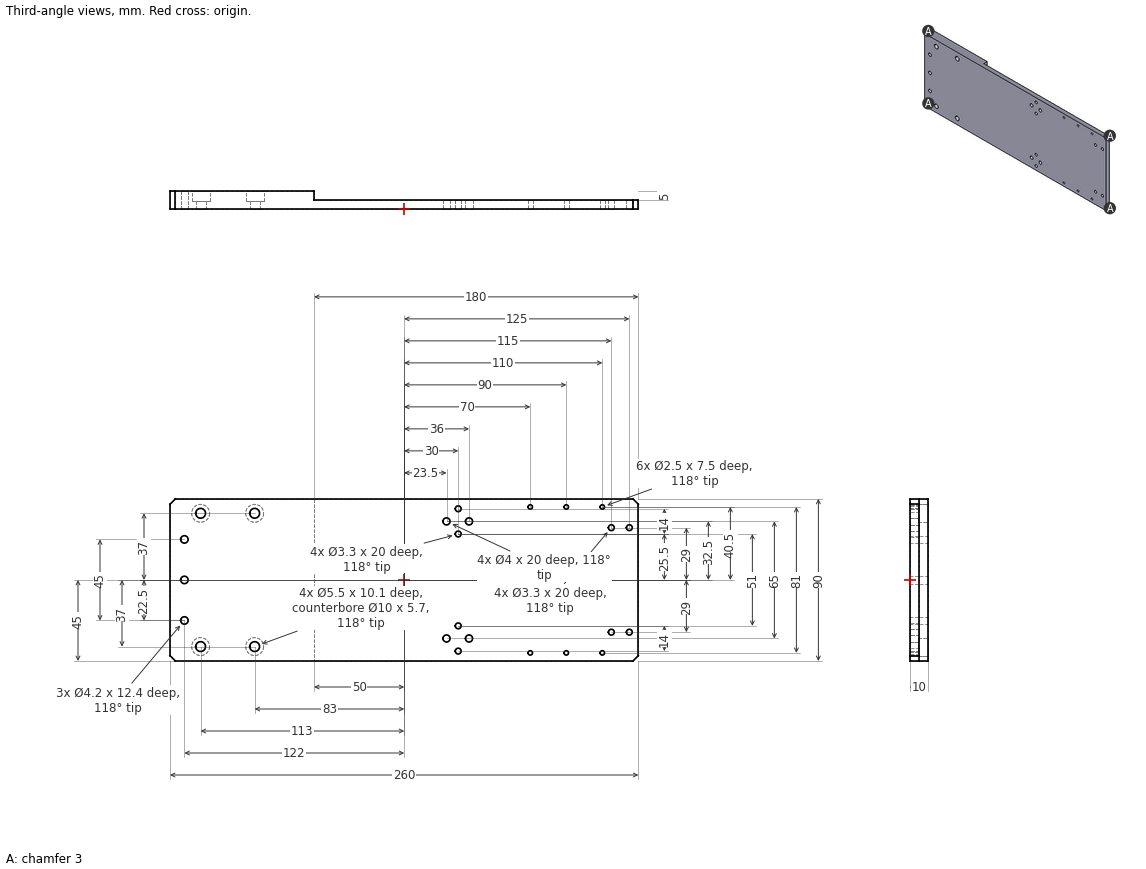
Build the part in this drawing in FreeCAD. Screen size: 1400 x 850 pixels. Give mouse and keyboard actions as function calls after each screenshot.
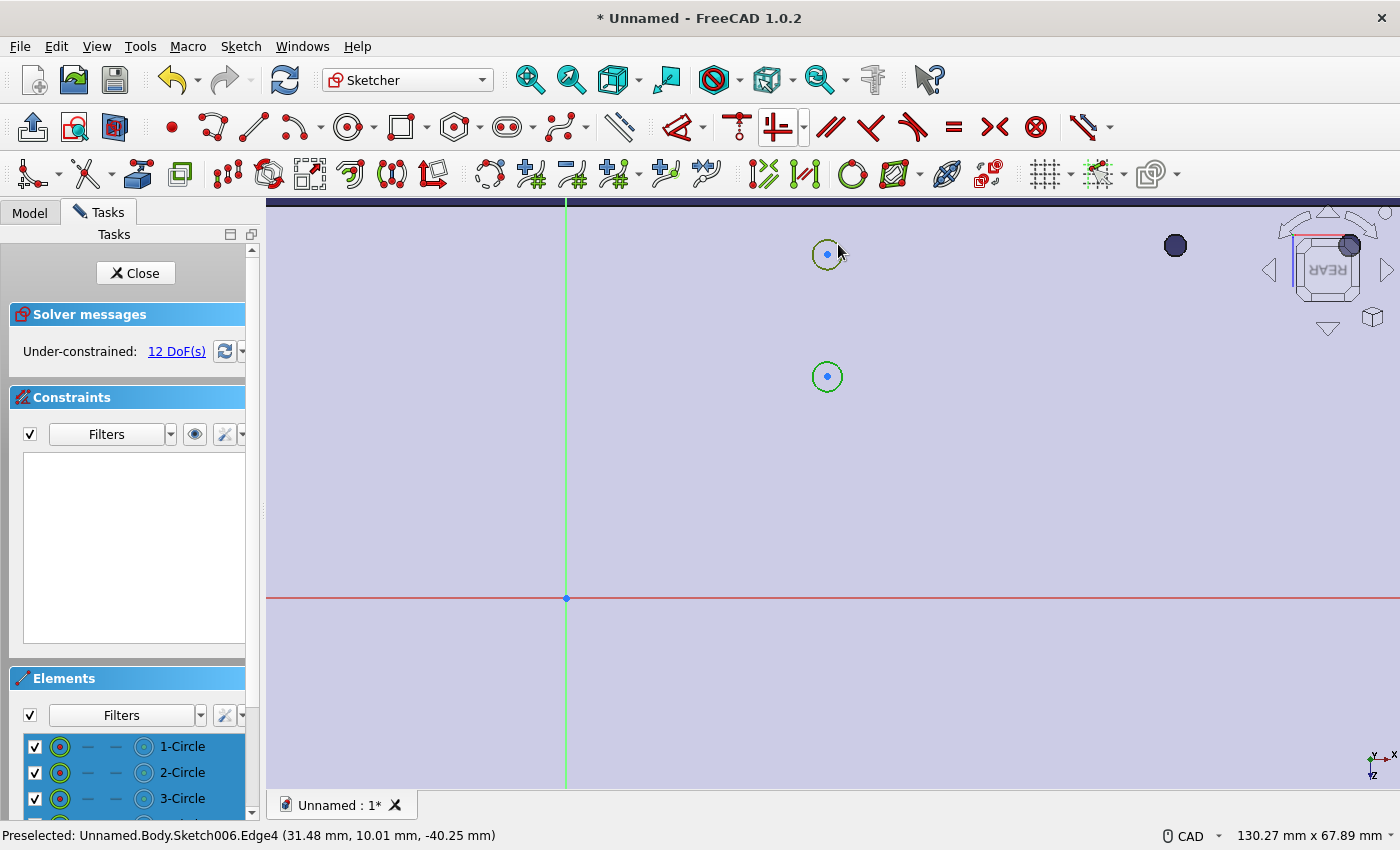
click(954, 128)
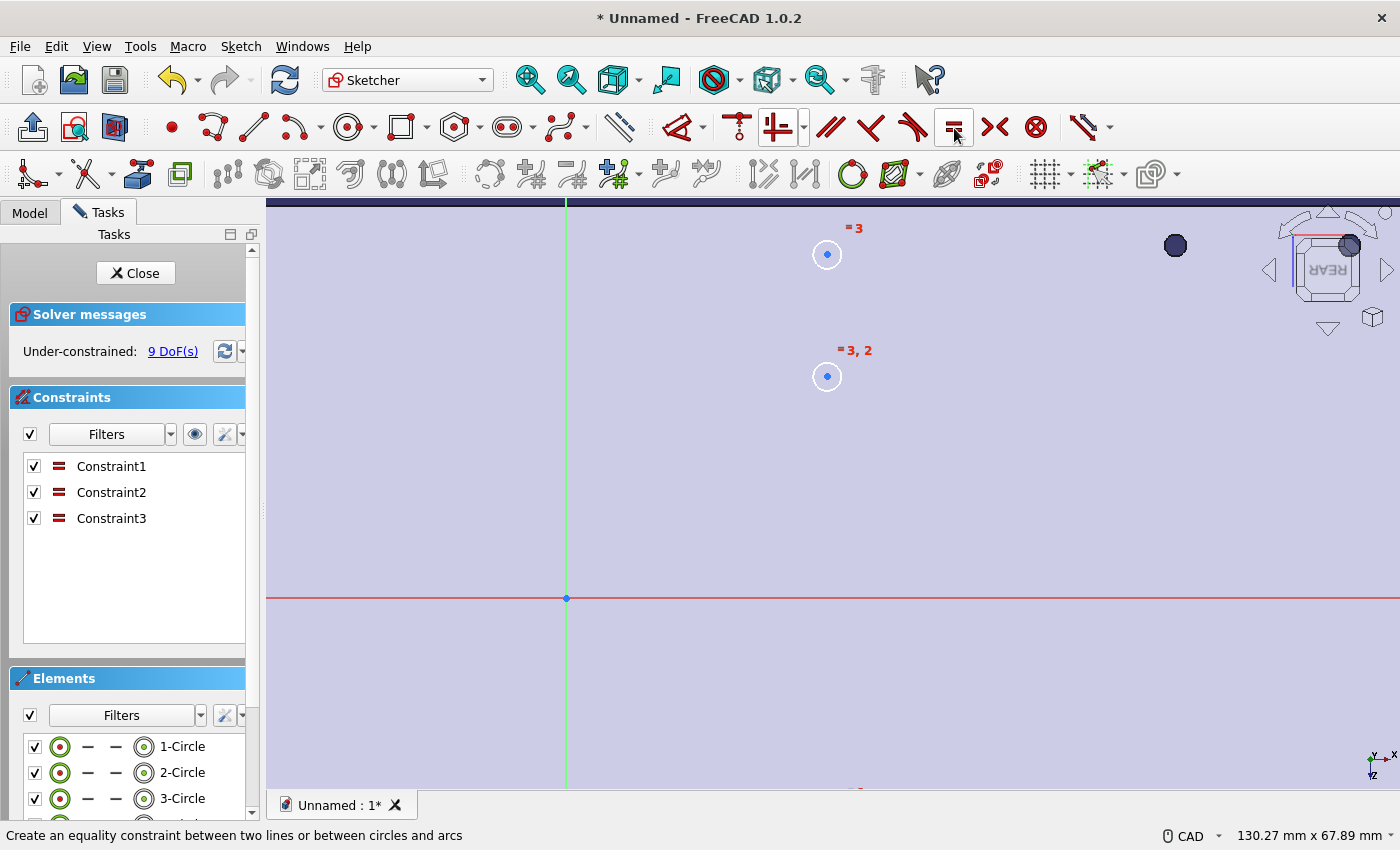
scroll(838, 366, down, 3)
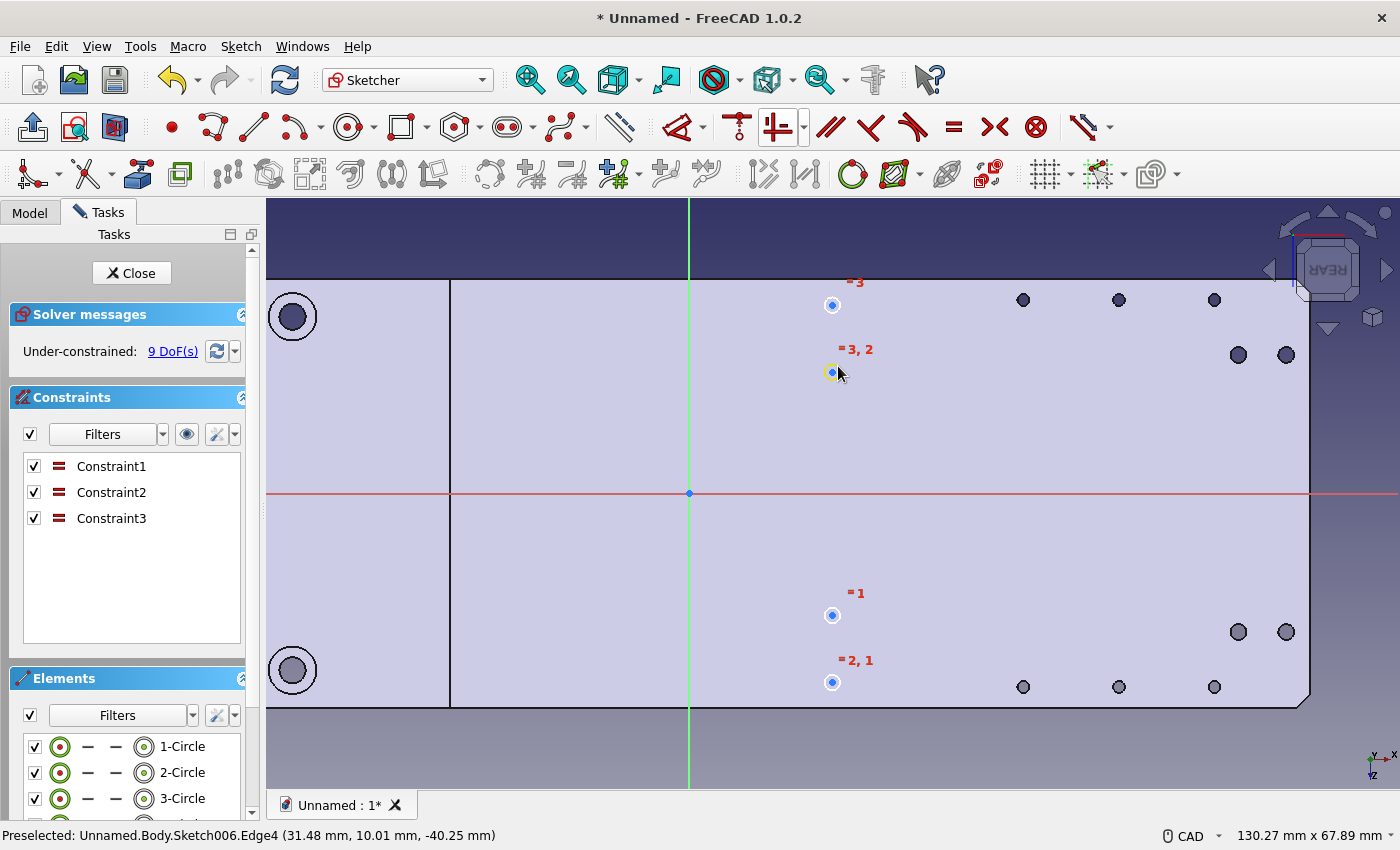
click(832, 615)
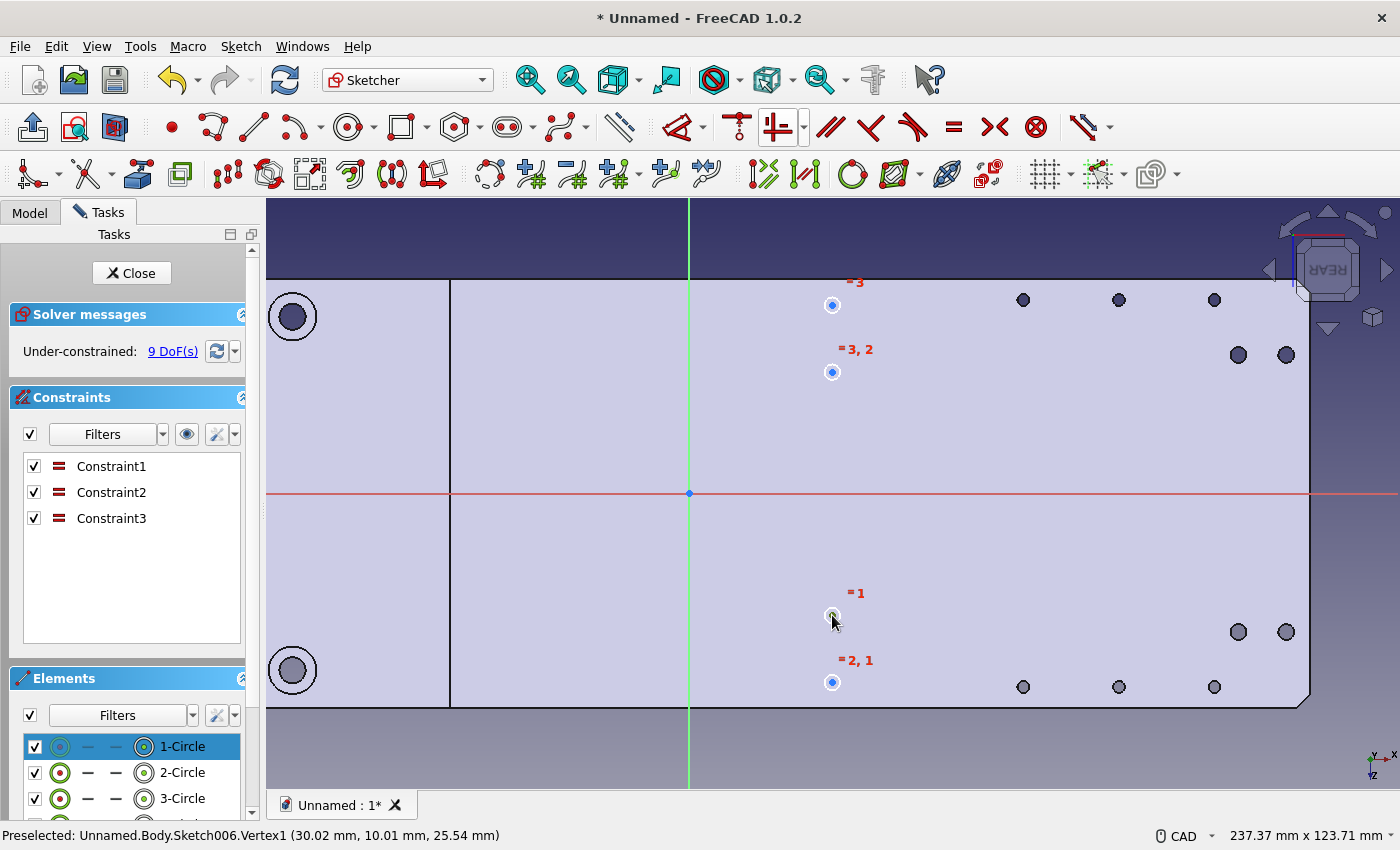
click(832, 683)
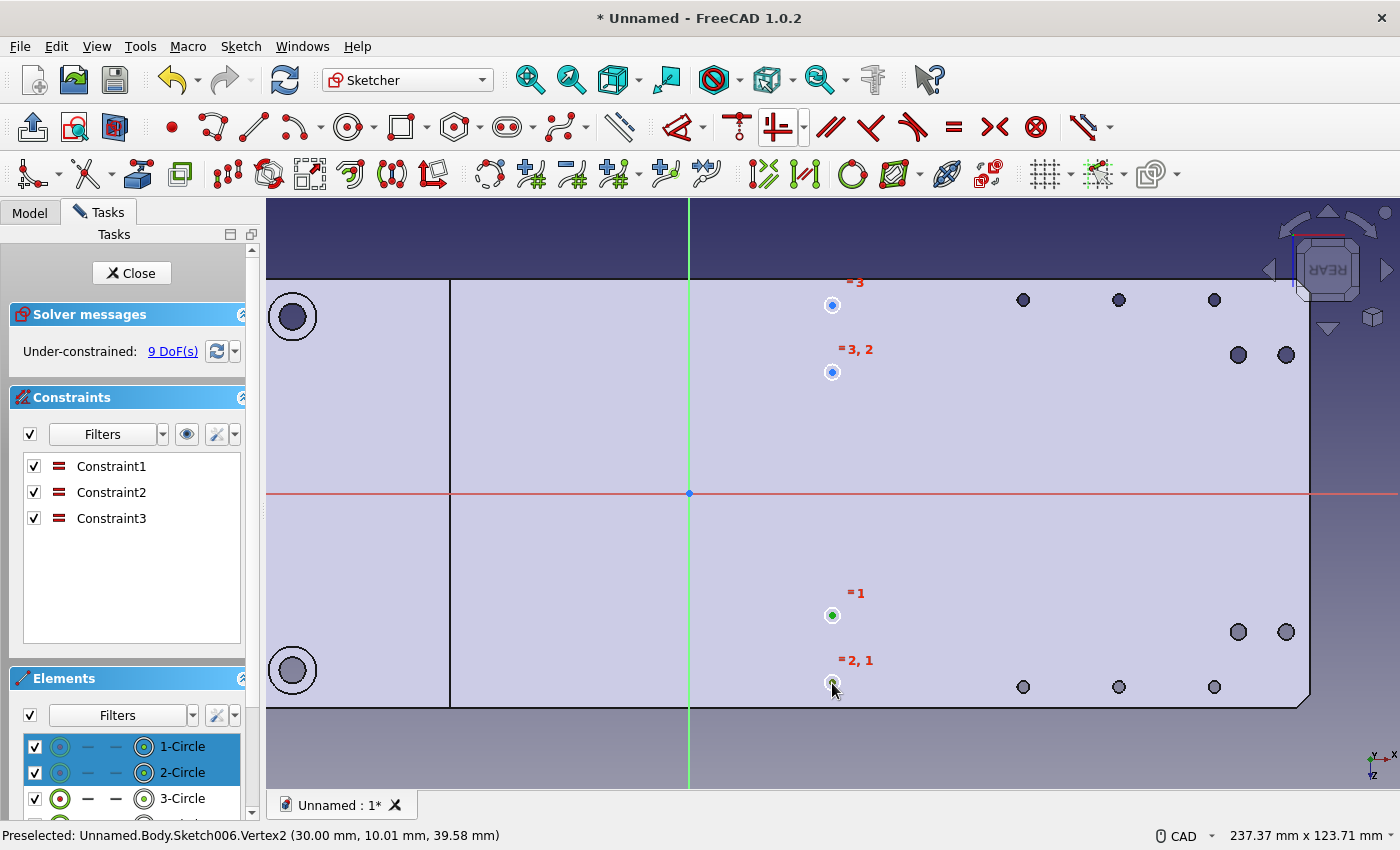
click(804, 128)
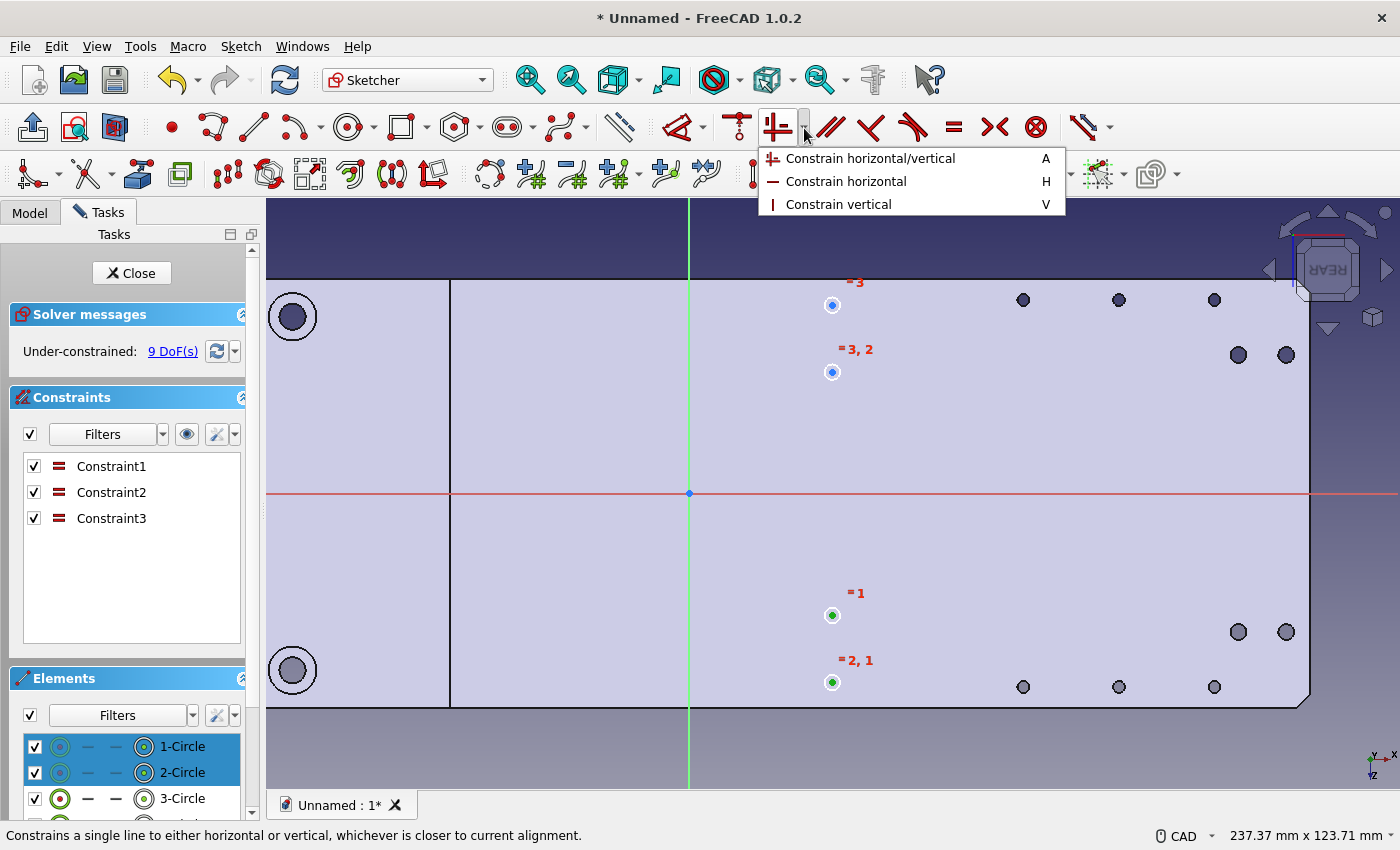
click(912, 204)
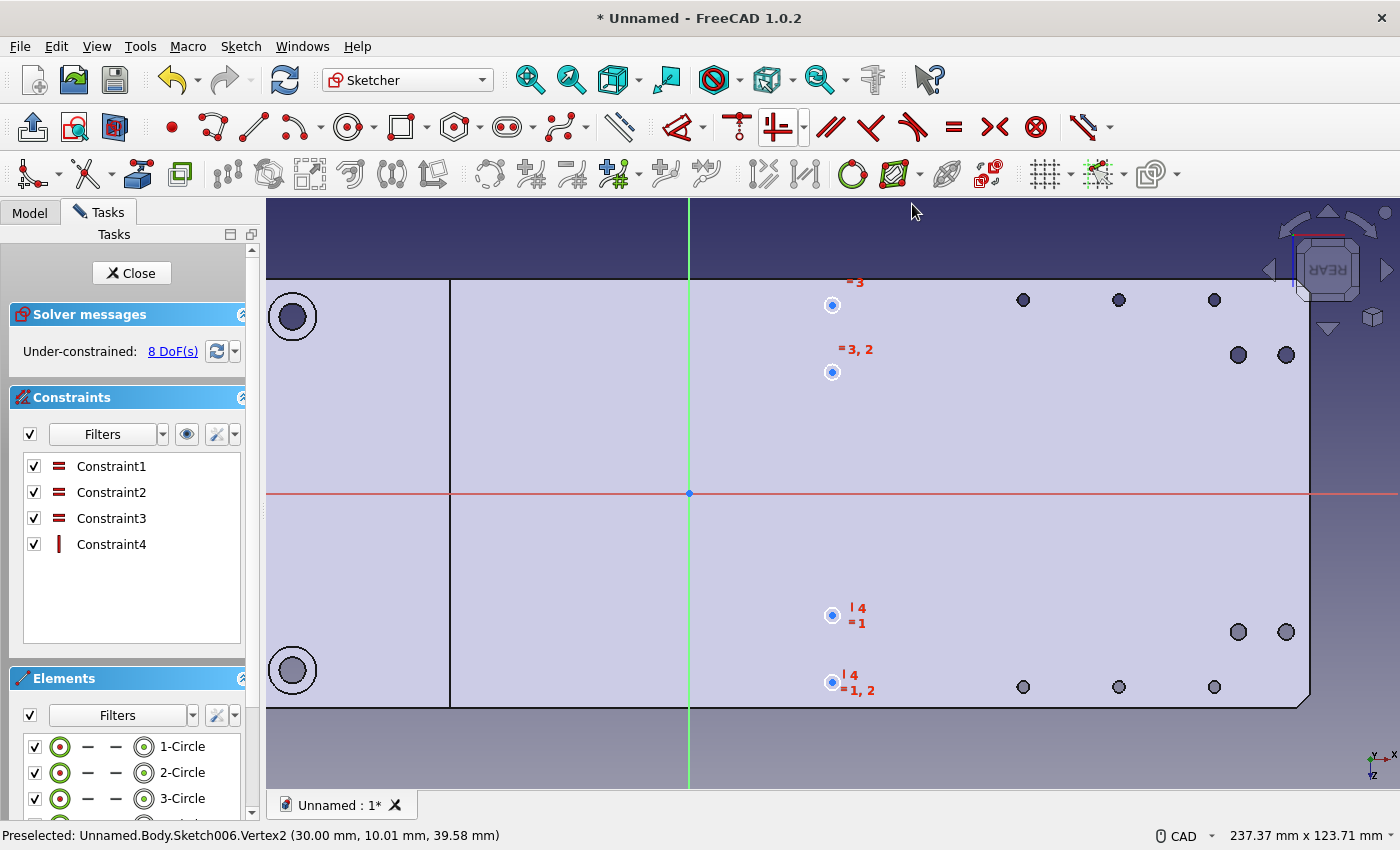
click(832, 615)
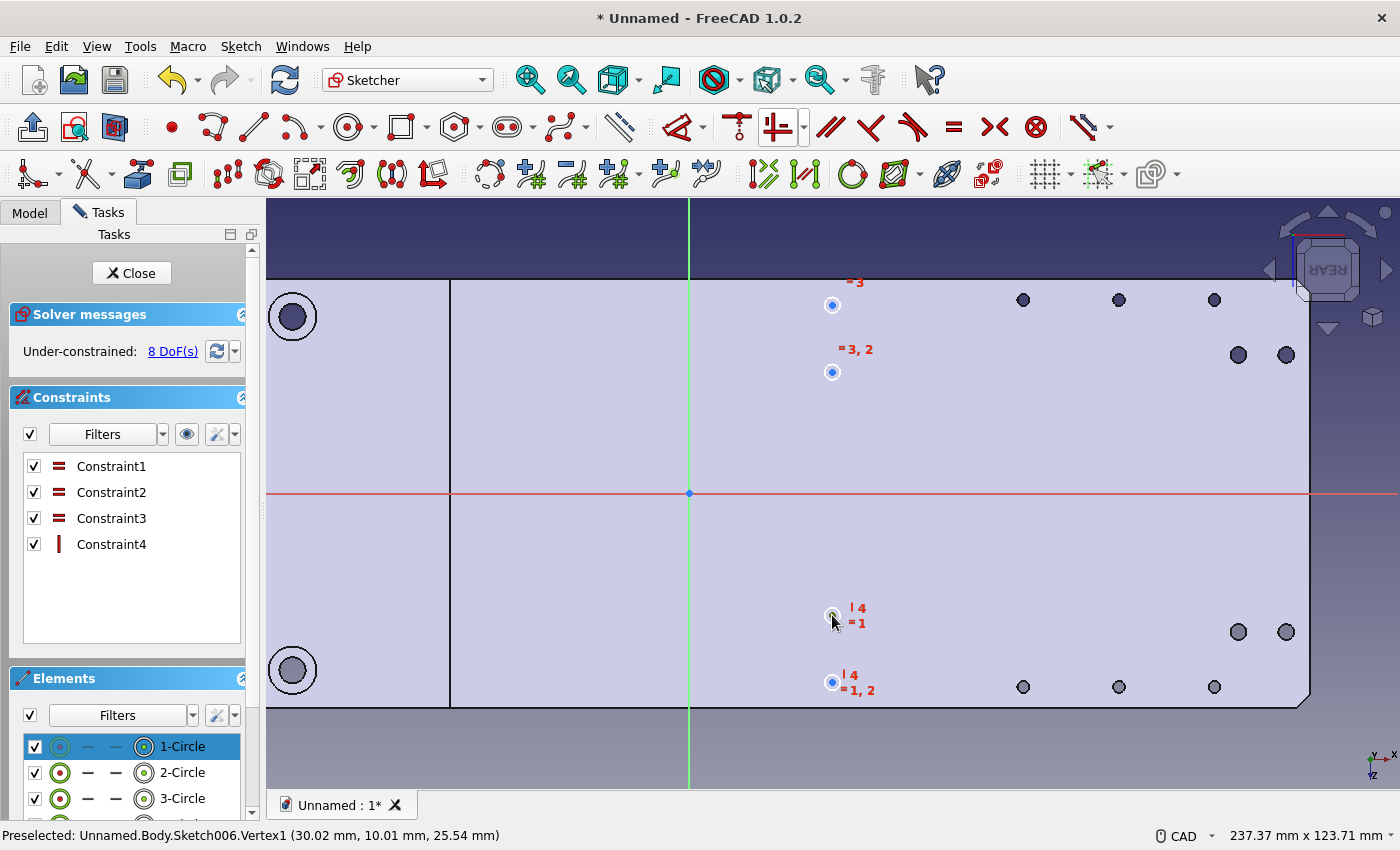
click(832, 372)